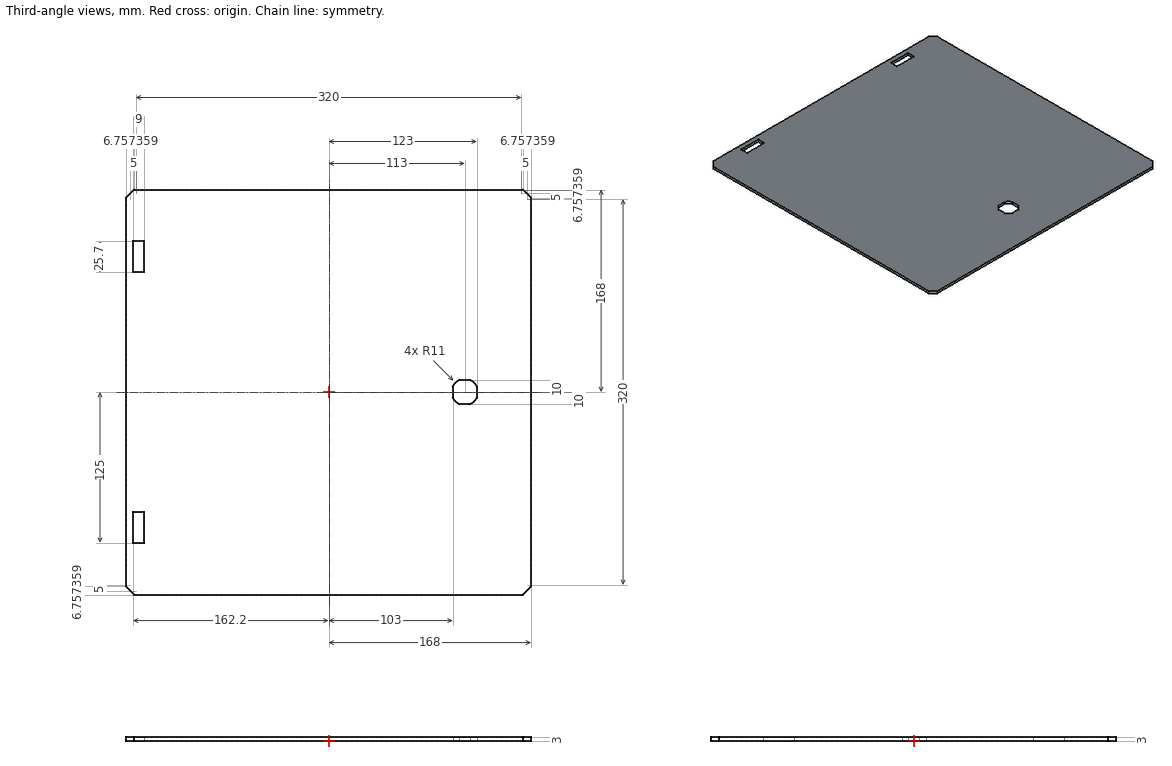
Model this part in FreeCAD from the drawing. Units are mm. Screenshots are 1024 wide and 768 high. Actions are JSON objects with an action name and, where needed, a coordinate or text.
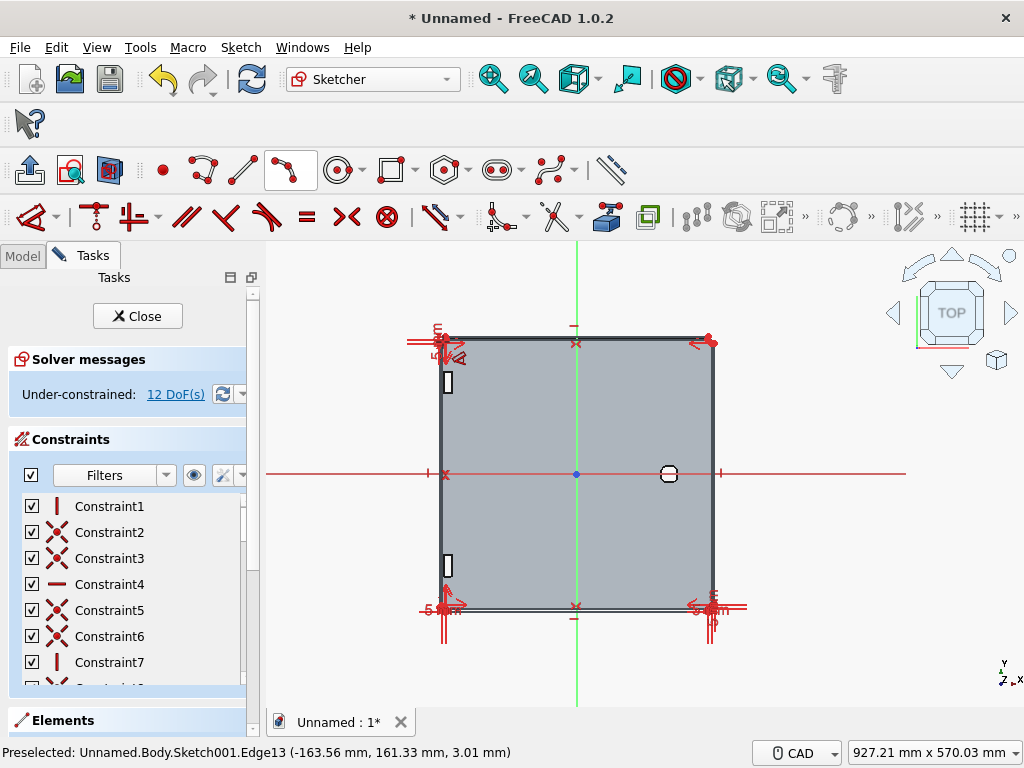
{"action": "scroll", "coordinate": [709, 341], "scroll_direction": "up", "scroll_amount": 12}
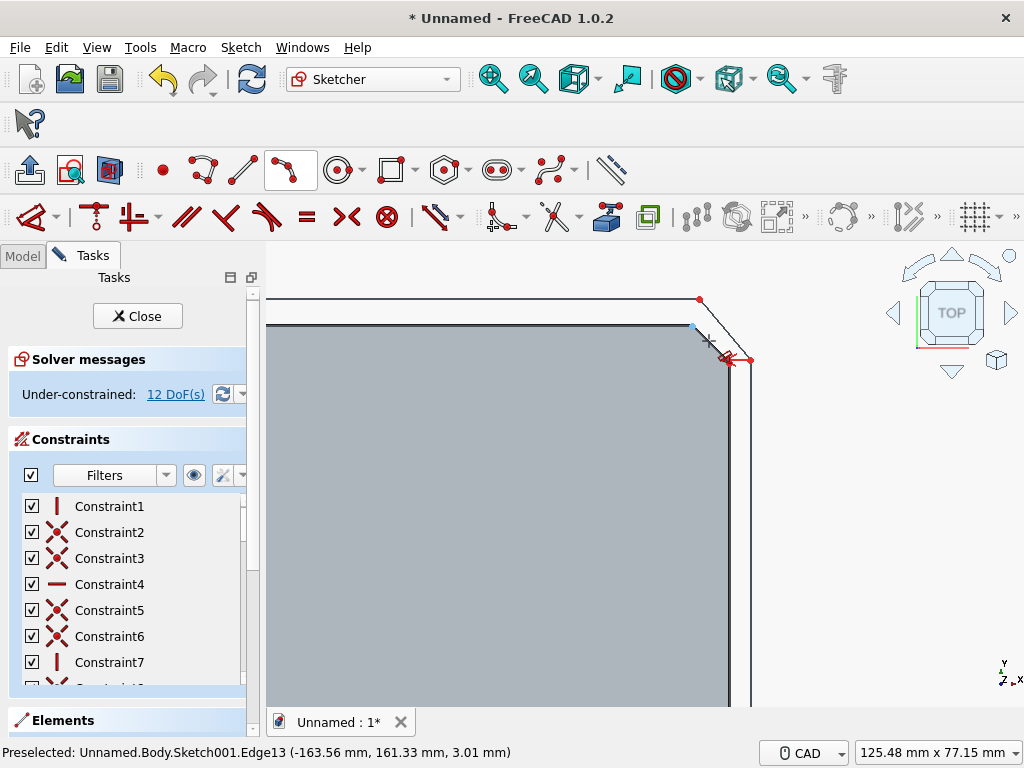
{"action": "left_click", "coordinate": [702, 336]}
{"action": "left_click", "coordinate": [722, 289]}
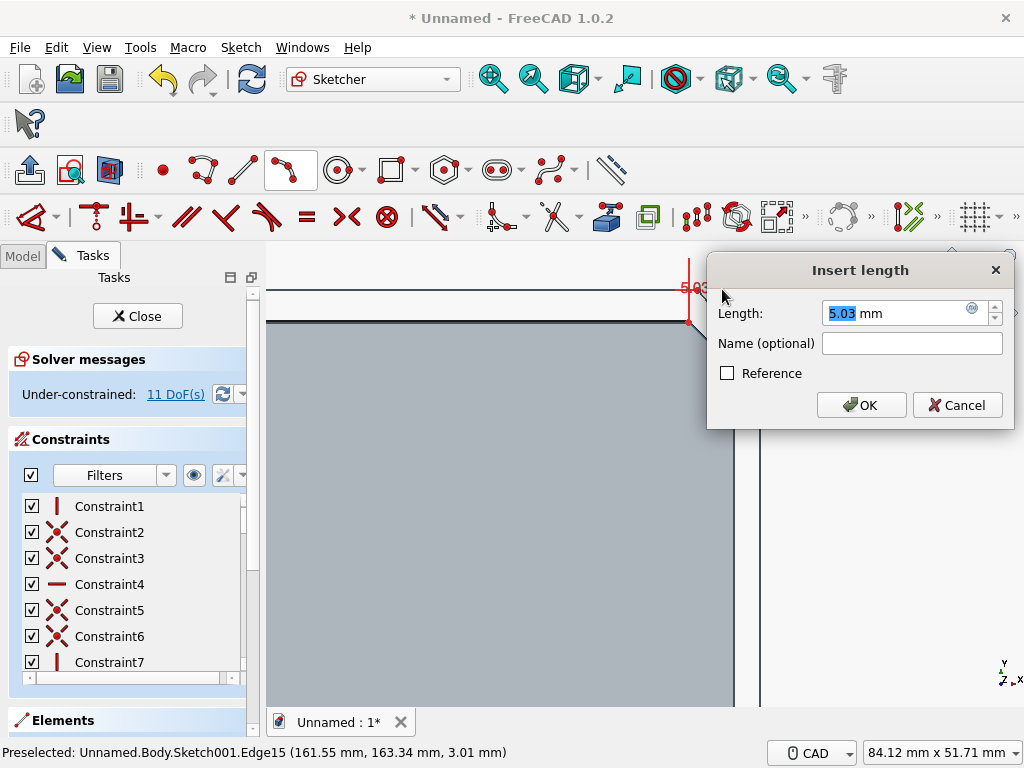
{"action": "type", "text": "5"}
{"action": "key", "text": "Return"}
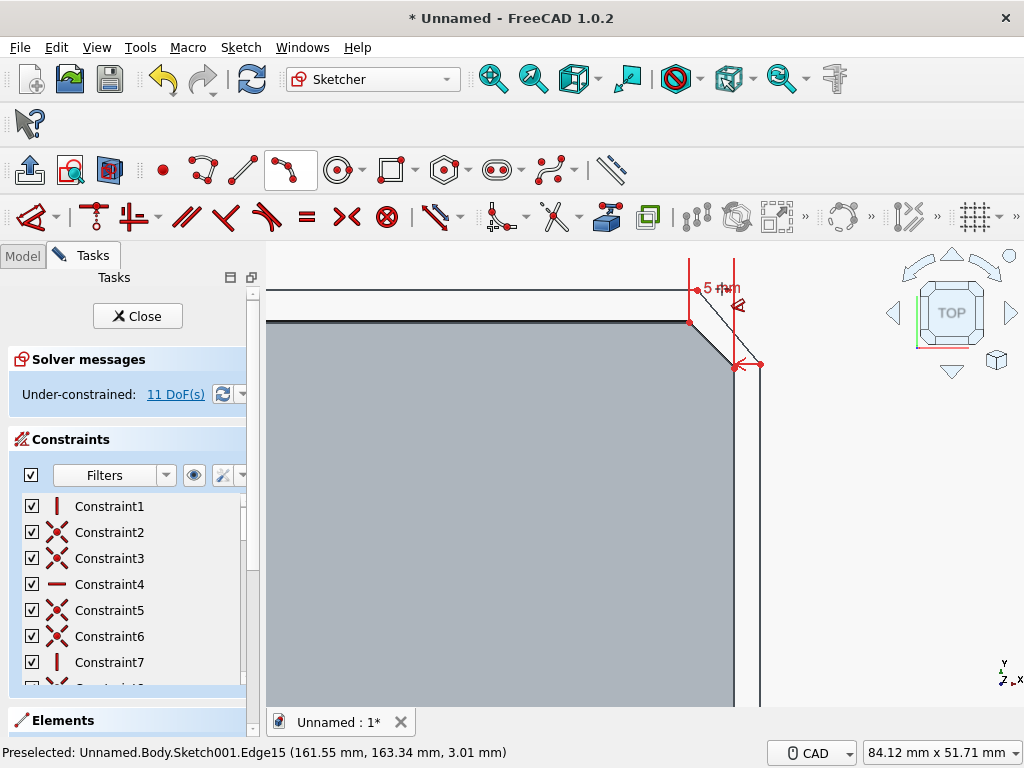
{"action": "left_click", "coordinate": [703, 336]}
{"action": "left_click", "coordinate": [768, 345]}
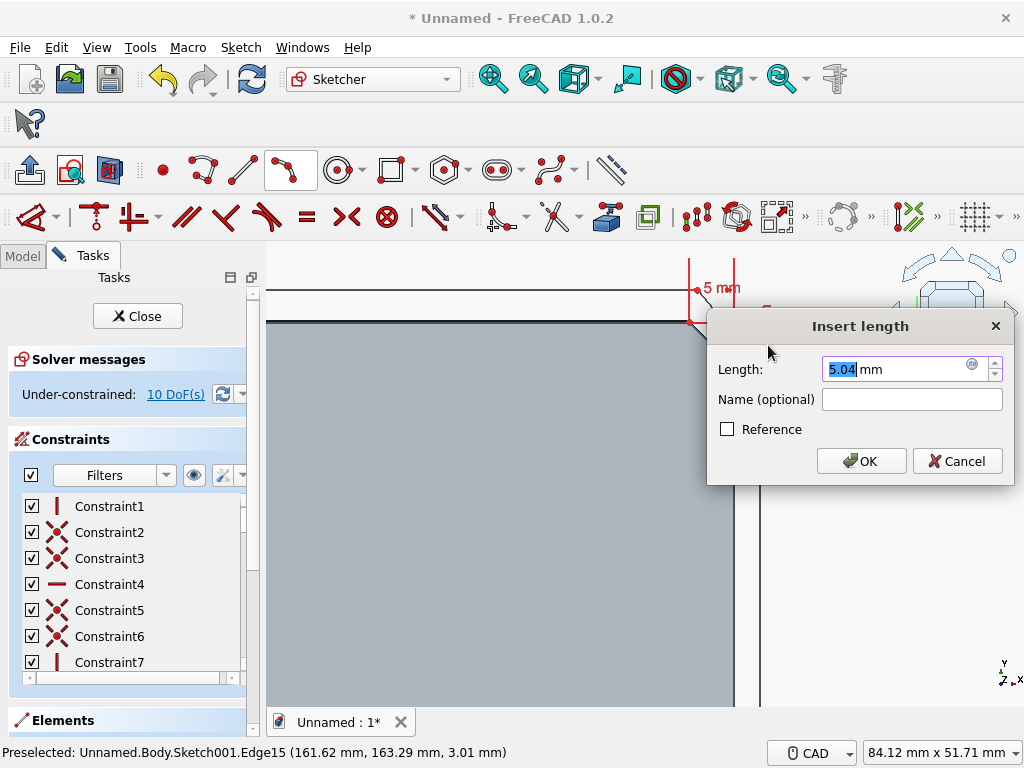
{"action": "type", "text": "5"}
{"action": "key", "text": "Return"}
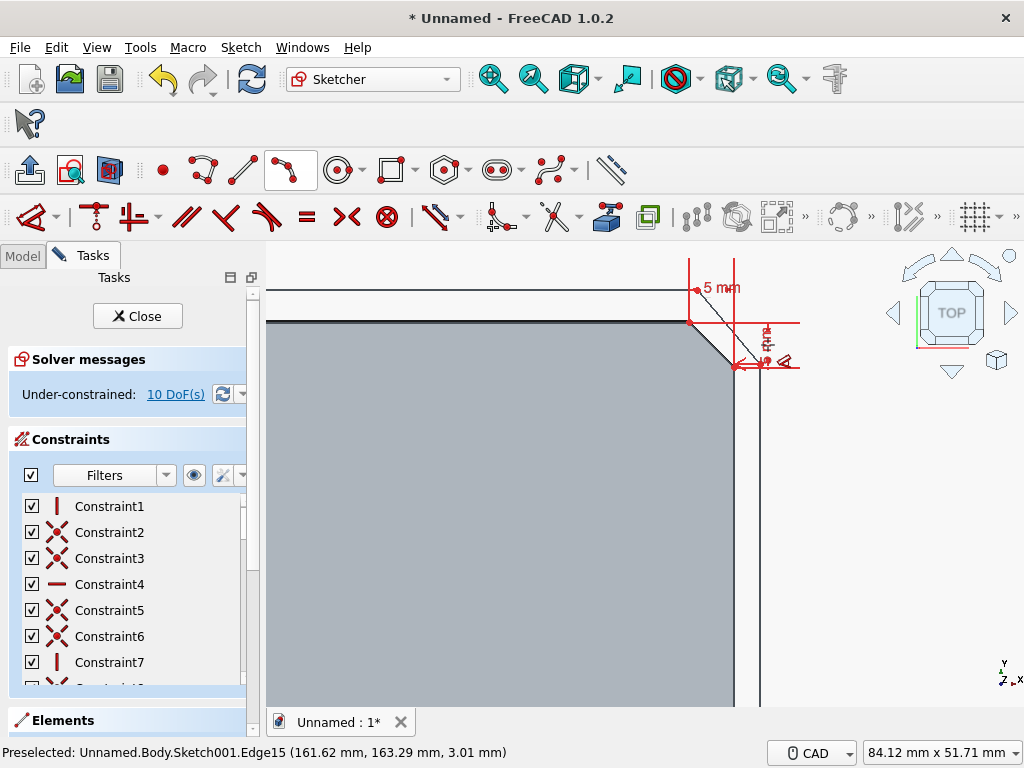
{"action": "scroll", "coordinate": [709, 341], "scroll_direction": "down", "scroll_amount": 12}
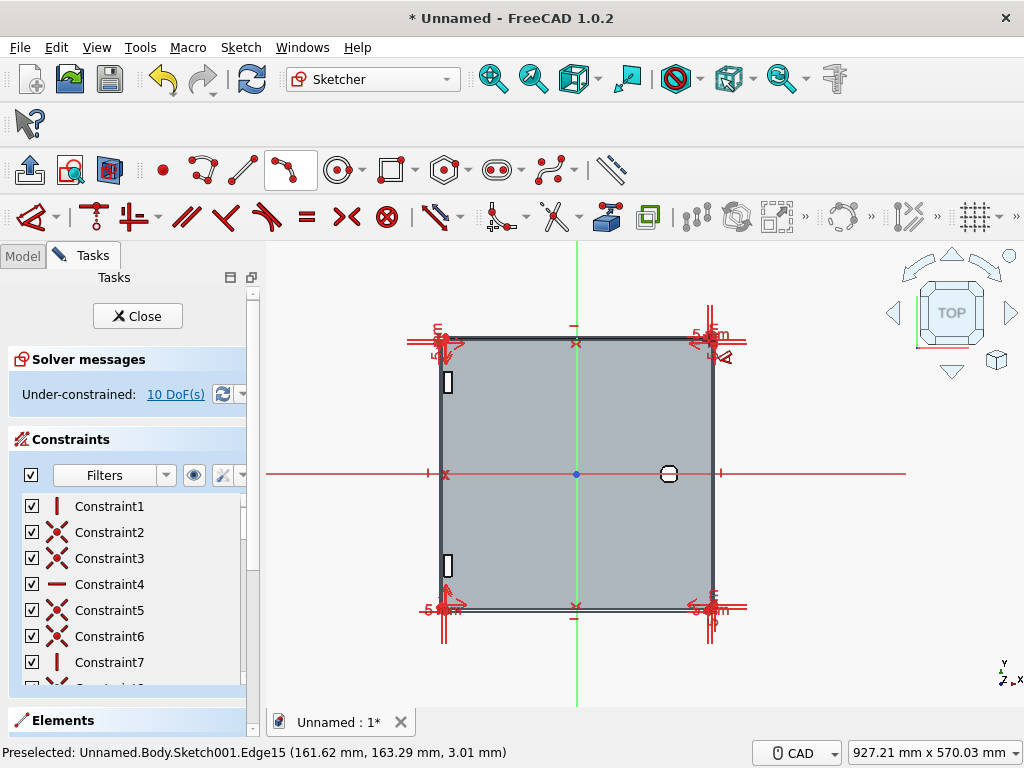
{"action": "scroll", "coordinate": [629, 609], "scroll_direction": "up", "scroll_amount": 8}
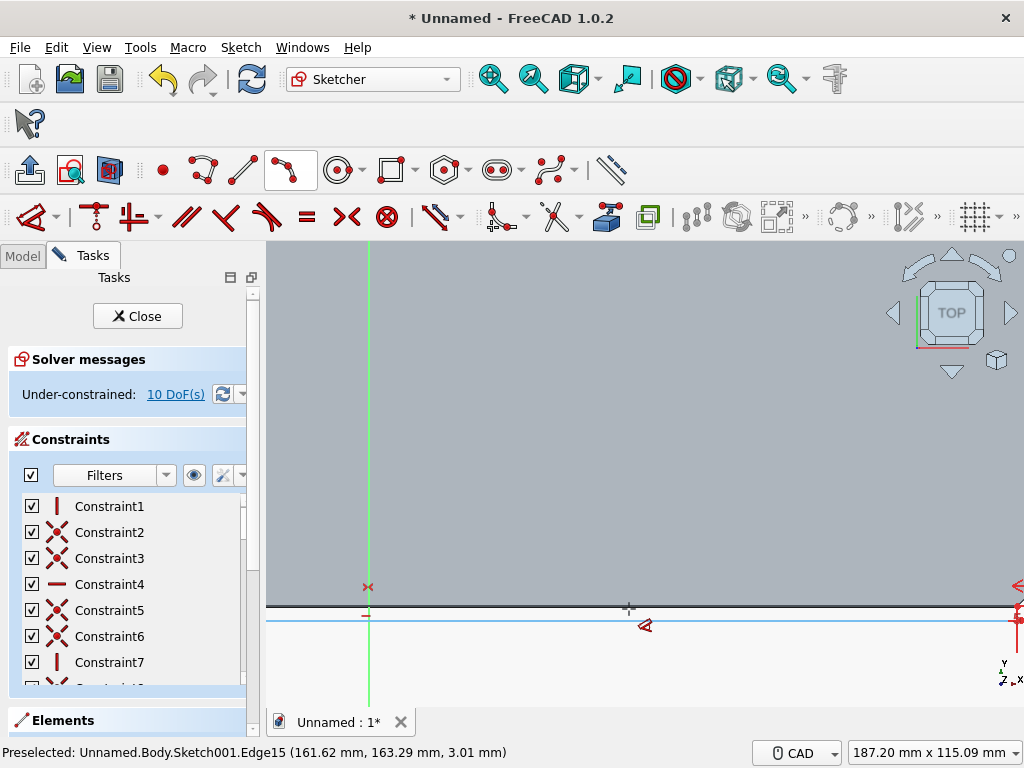
{"action": "left_click", "coordinate": [628, 606]}
{"action": "left_click", "coordinate": [576, 640]}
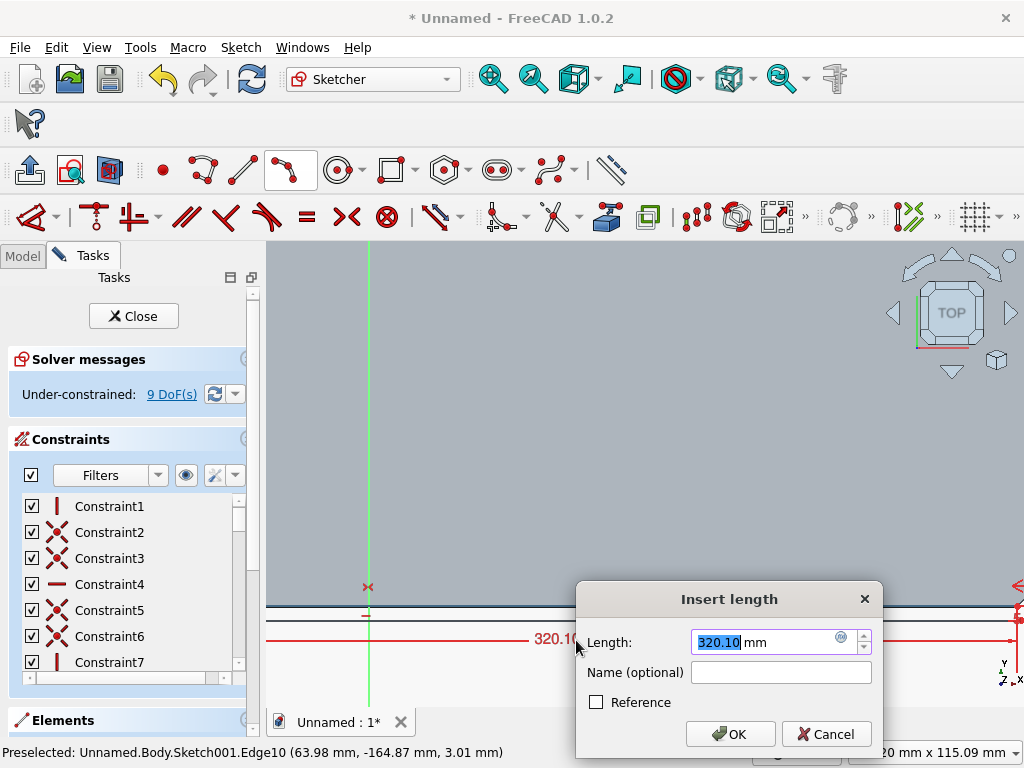
{"action": "type", "text": "320"}
{"action": "key", "text": "Return"}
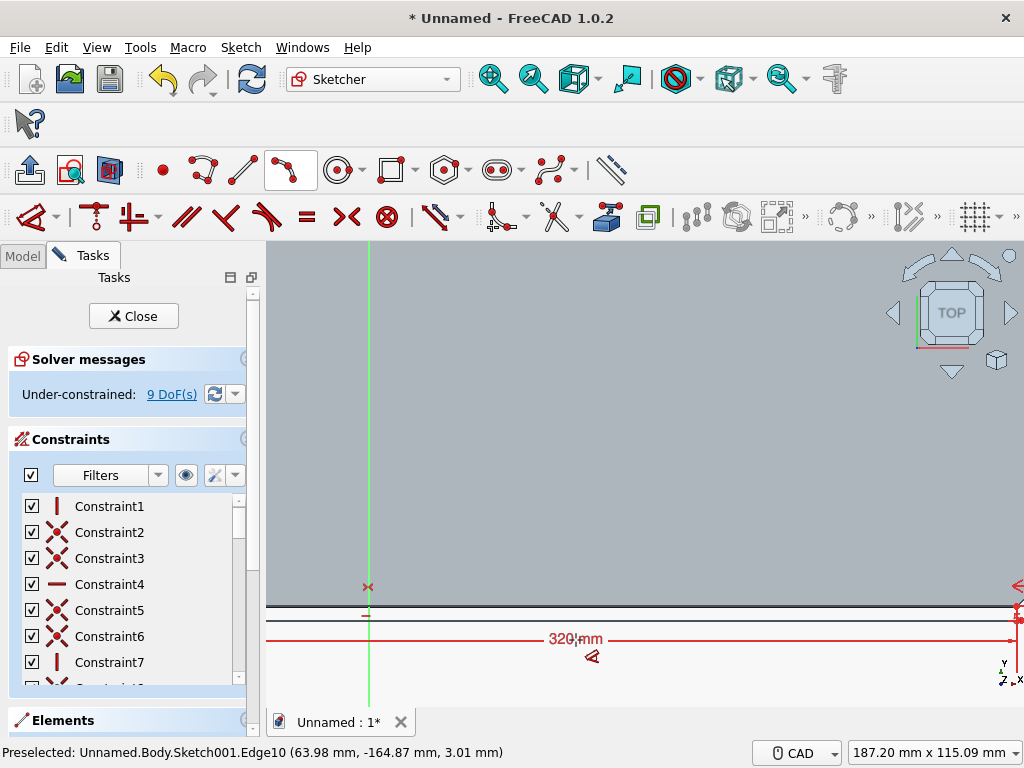
{"action": "scroll", "coordinate": [629, 609], "scroll_direction": "down", "scroll_amount": 8}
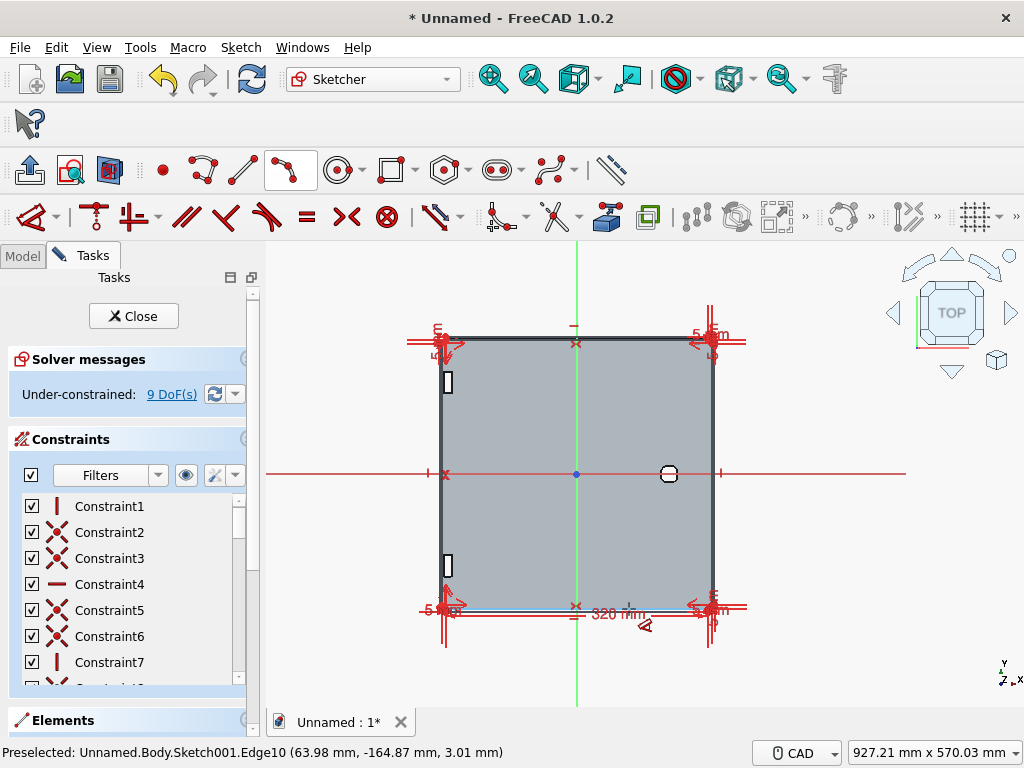
{"action": "scroll", "coordinate": [442, 527], "scroll_direction": "up", "scroll_amount": 9}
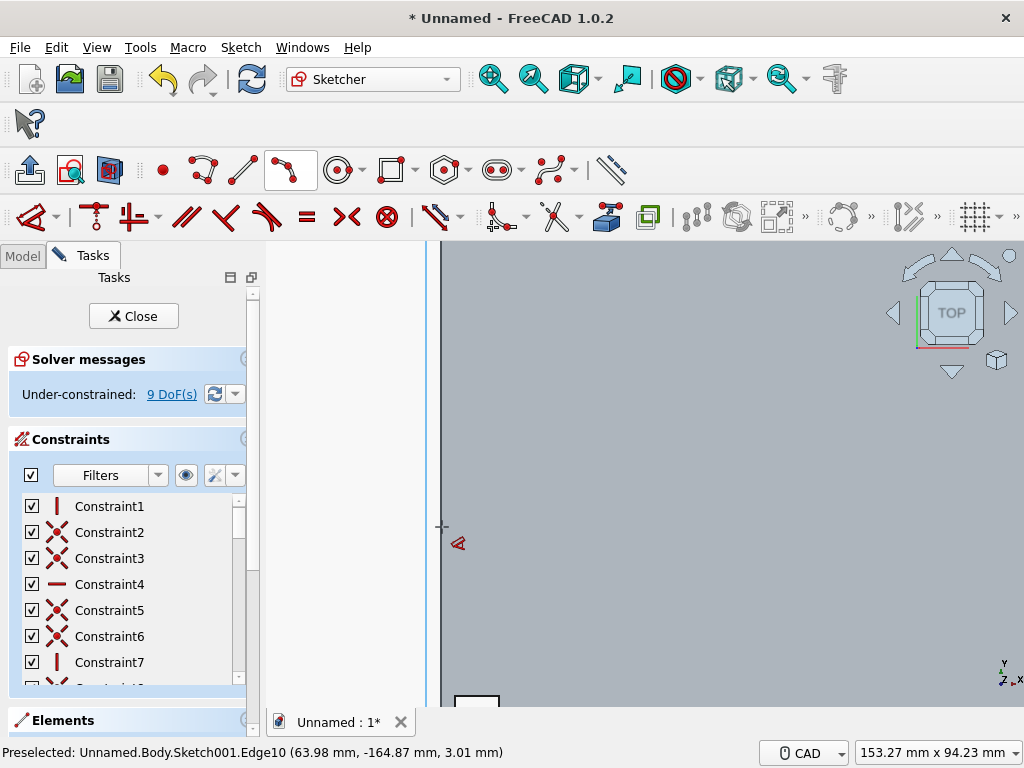
{"action": "left_click", "coordinate": [441, 521]}
{"action": "left_click", "coordinate": [407, 474]}